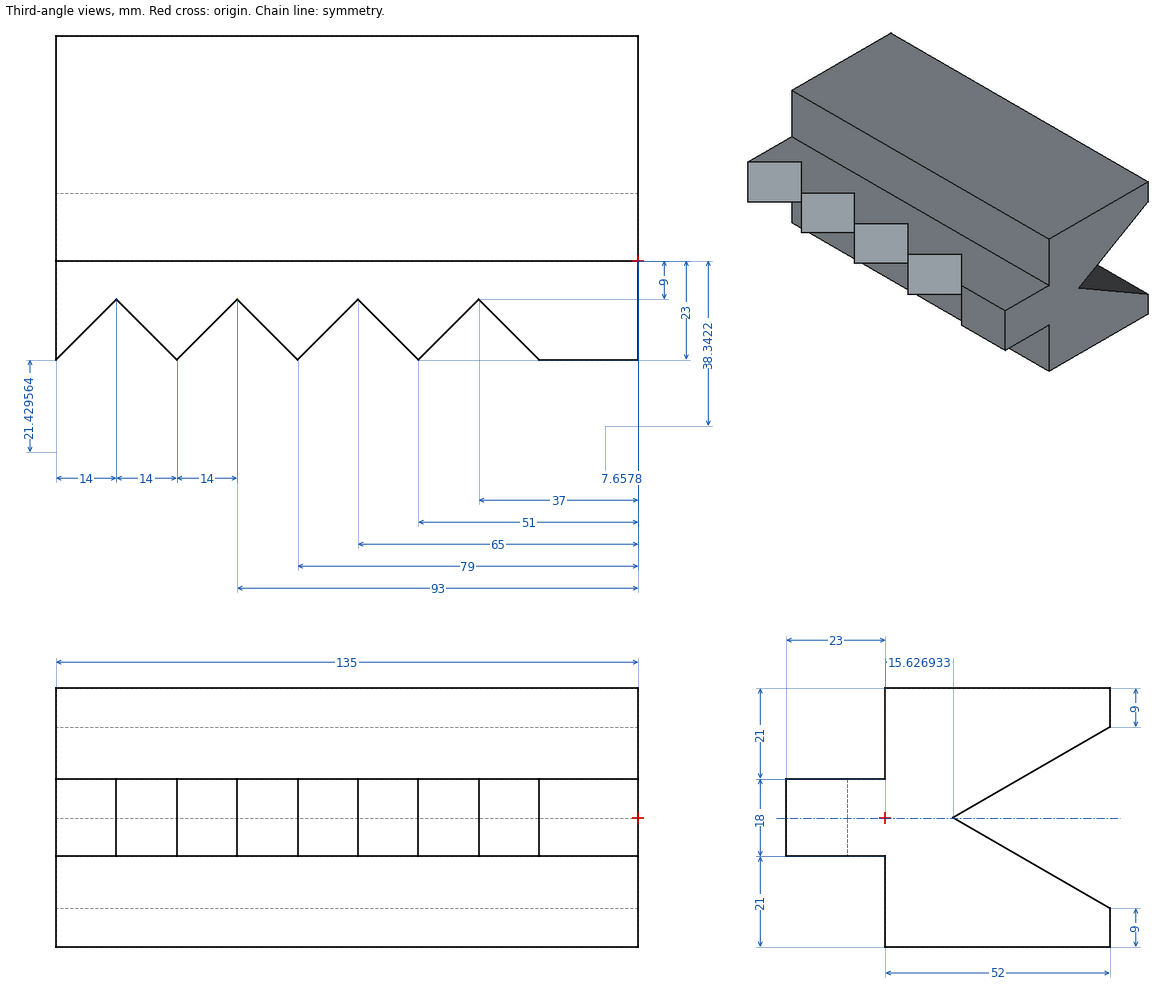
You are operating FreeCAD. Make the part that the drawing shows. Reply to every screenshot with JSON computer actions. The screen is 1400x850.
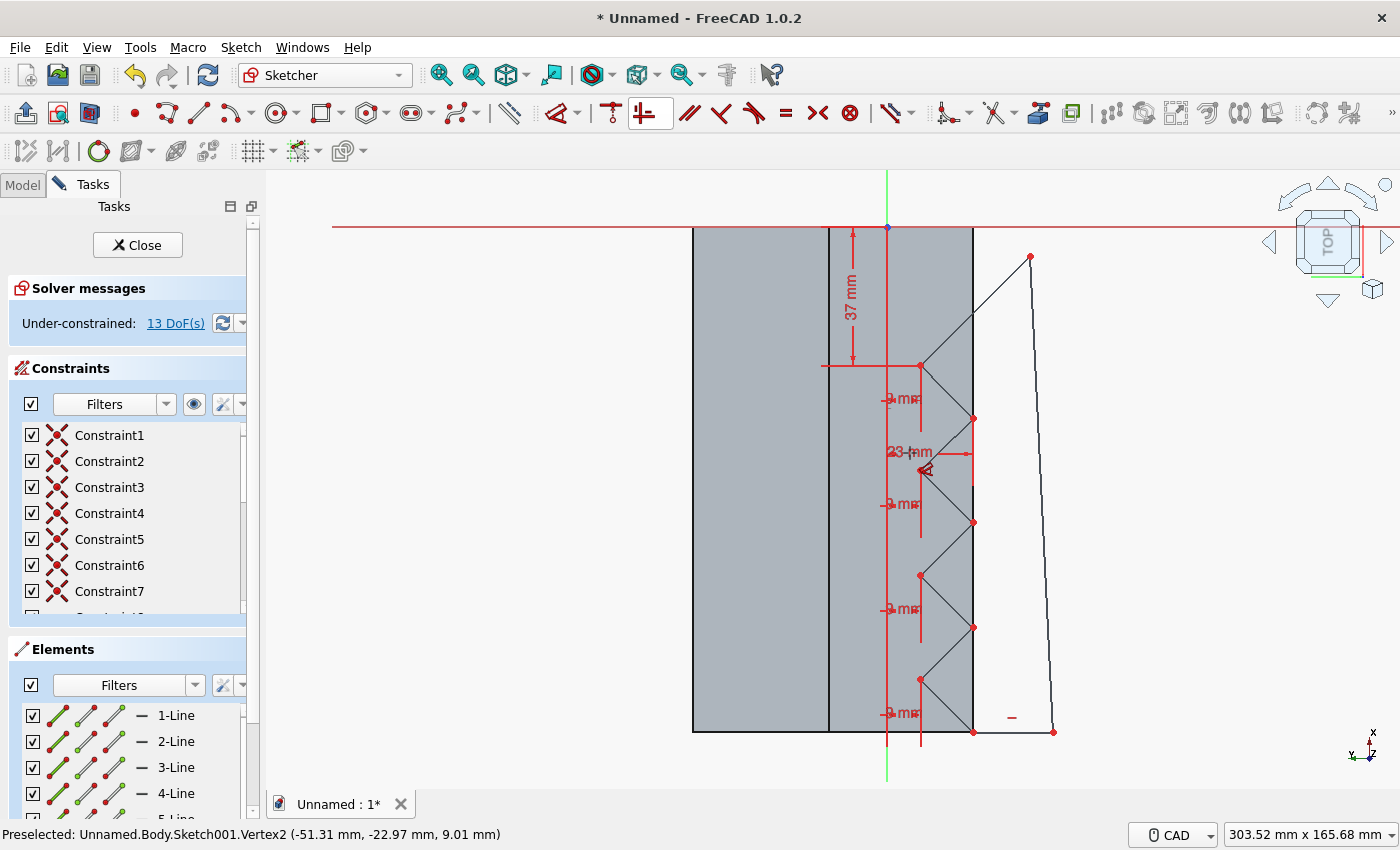
{"action": "left_click", "coordinate": [973, 419]}
{"action": "left_click", "coordinate": [853, 323]}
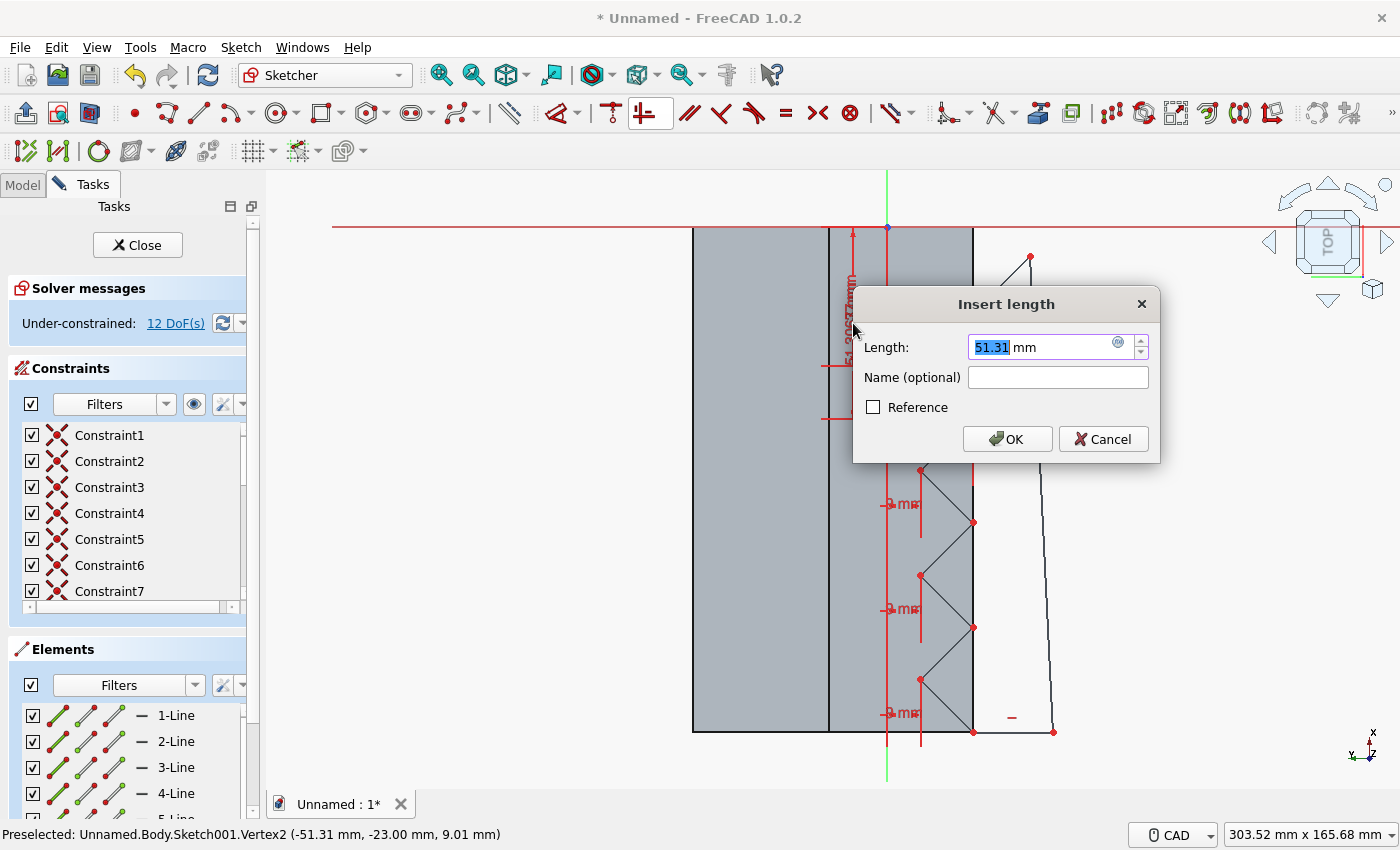
{"action": "type", "text": "51"}
{"action": "key", "text": "Return"}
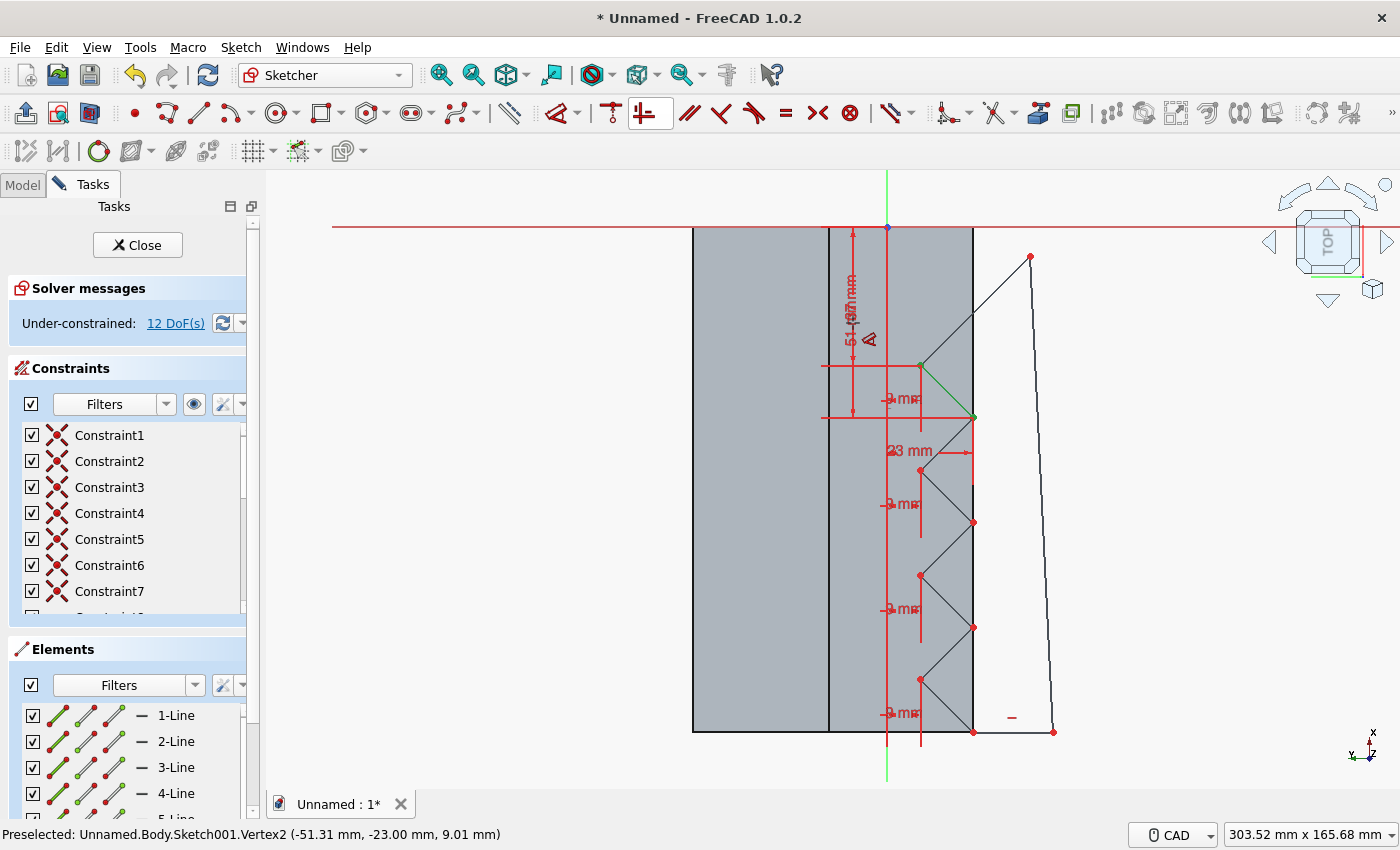
{"action": "left_click", "coordinate": [921, 471]}
{"action": "left_click", "coordinate": [853, 349]}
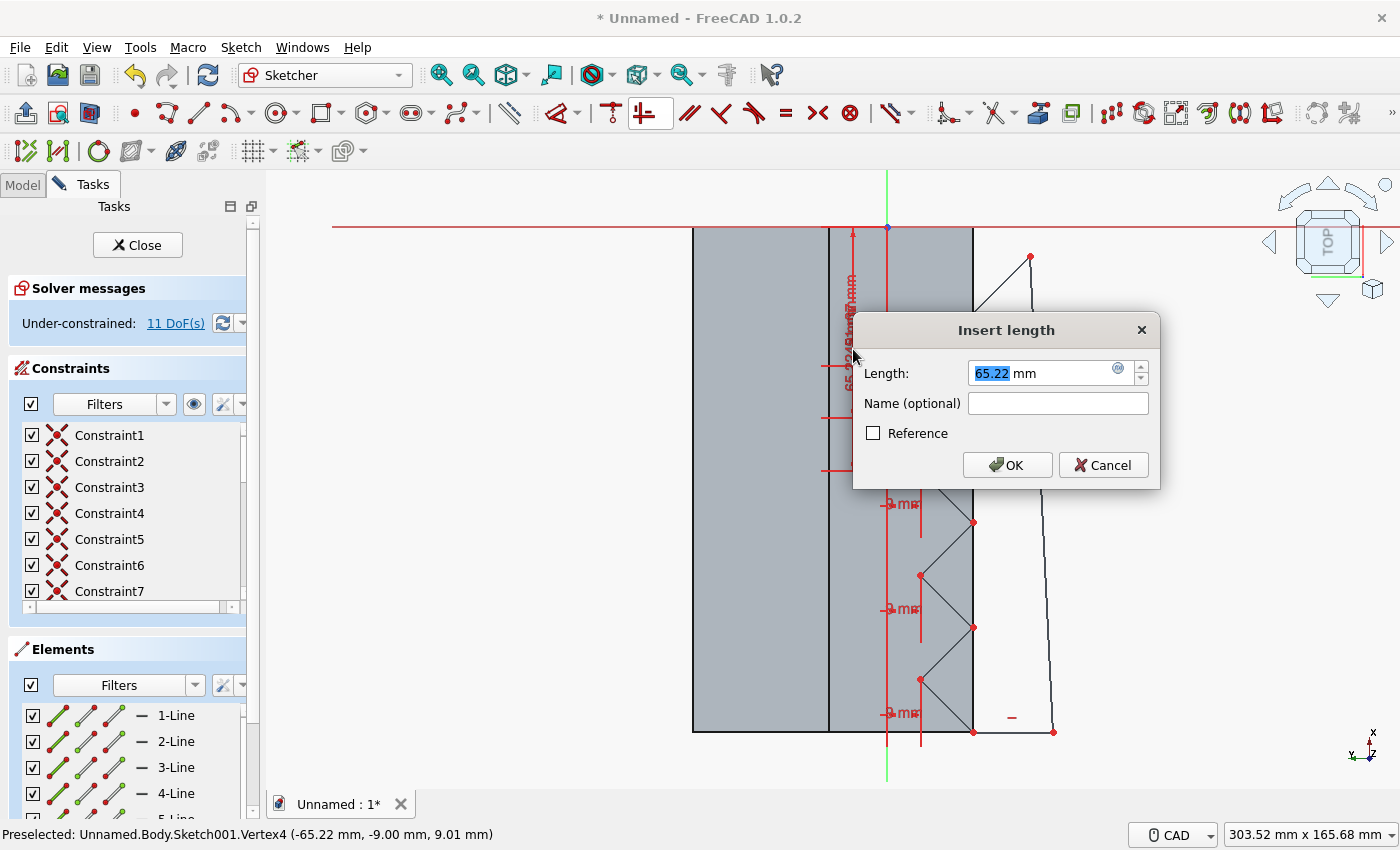
{"action": "type", "text": "65"}
{"action": "key", "text": "Return"}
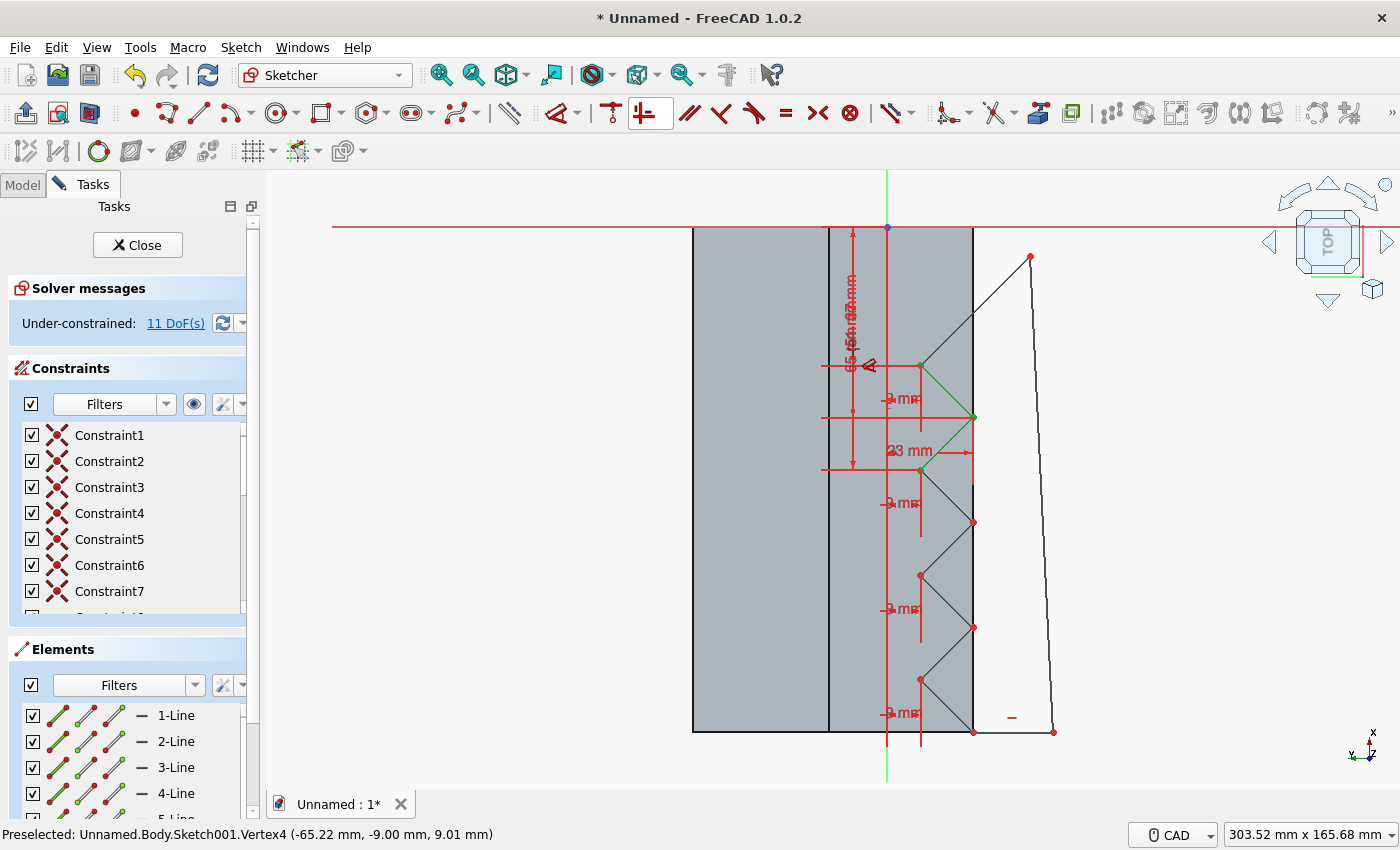
{"action": "left_click", "coordinate": [973, 523]}
{"action": "left_click", "coordinate": [910, 557]}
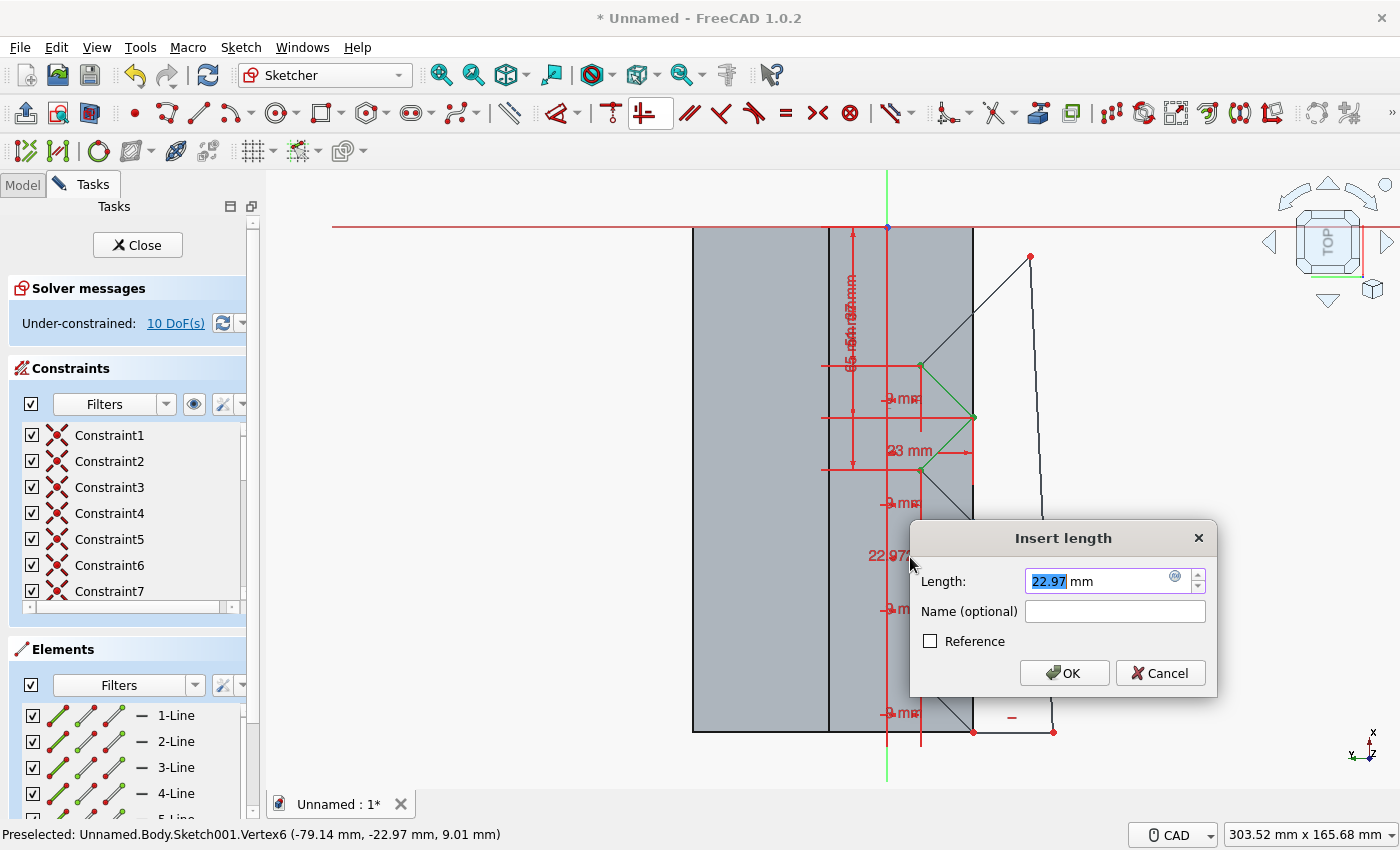
{"action": "type", "text": "23"}
{"action": "key", "text": "Return"}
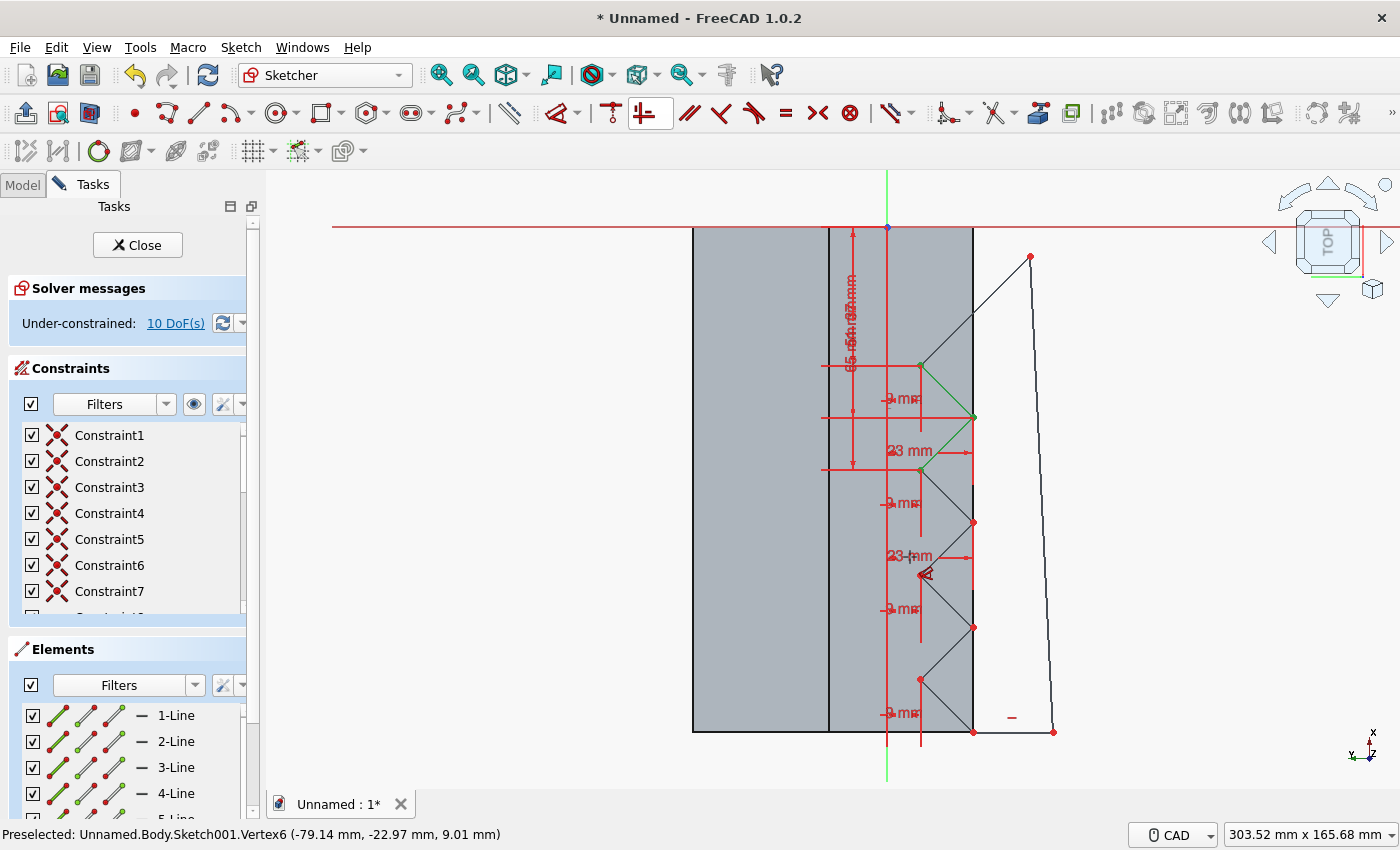
{"action": "left_click", "coordinate": [973, 523]}
{"action": "left_click", "coordinate": [853, 375]}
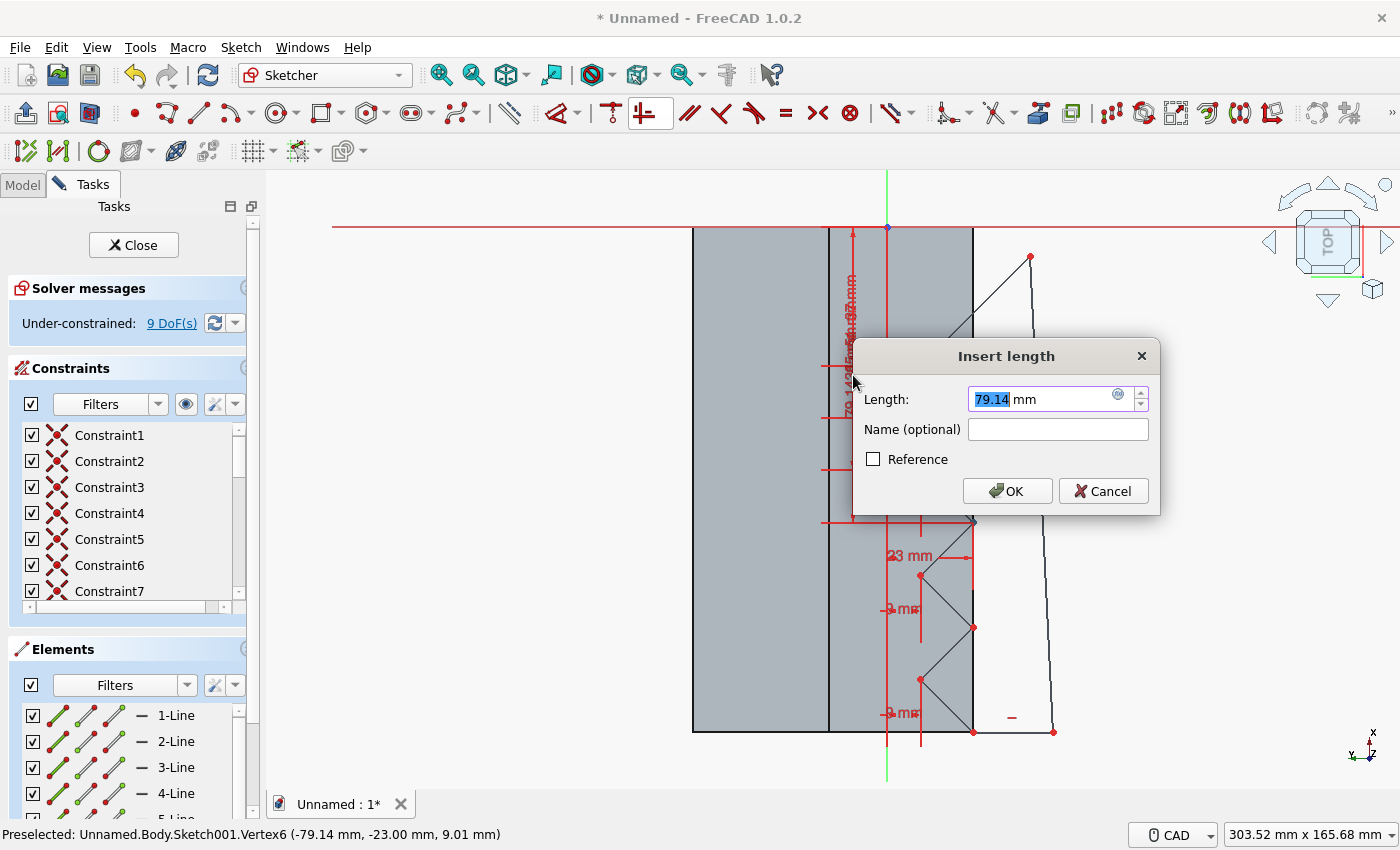
{"action": "type", "text": "79"}
{"action": "key", "text": "Return"}